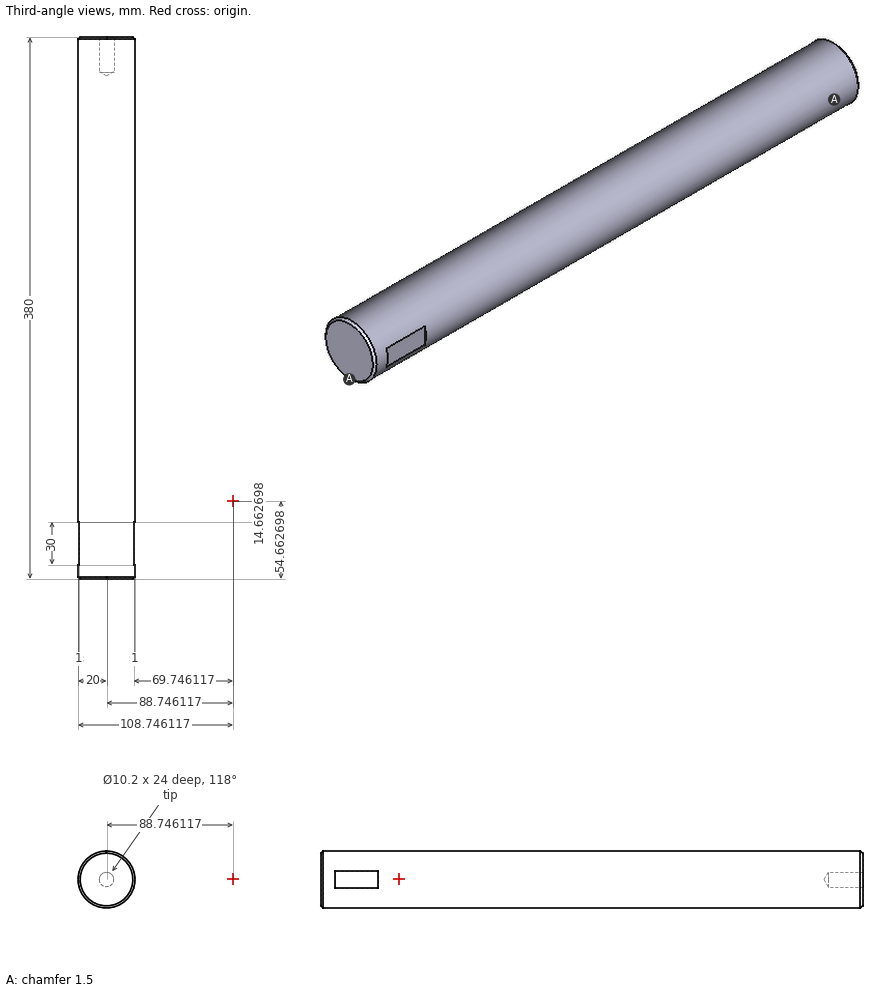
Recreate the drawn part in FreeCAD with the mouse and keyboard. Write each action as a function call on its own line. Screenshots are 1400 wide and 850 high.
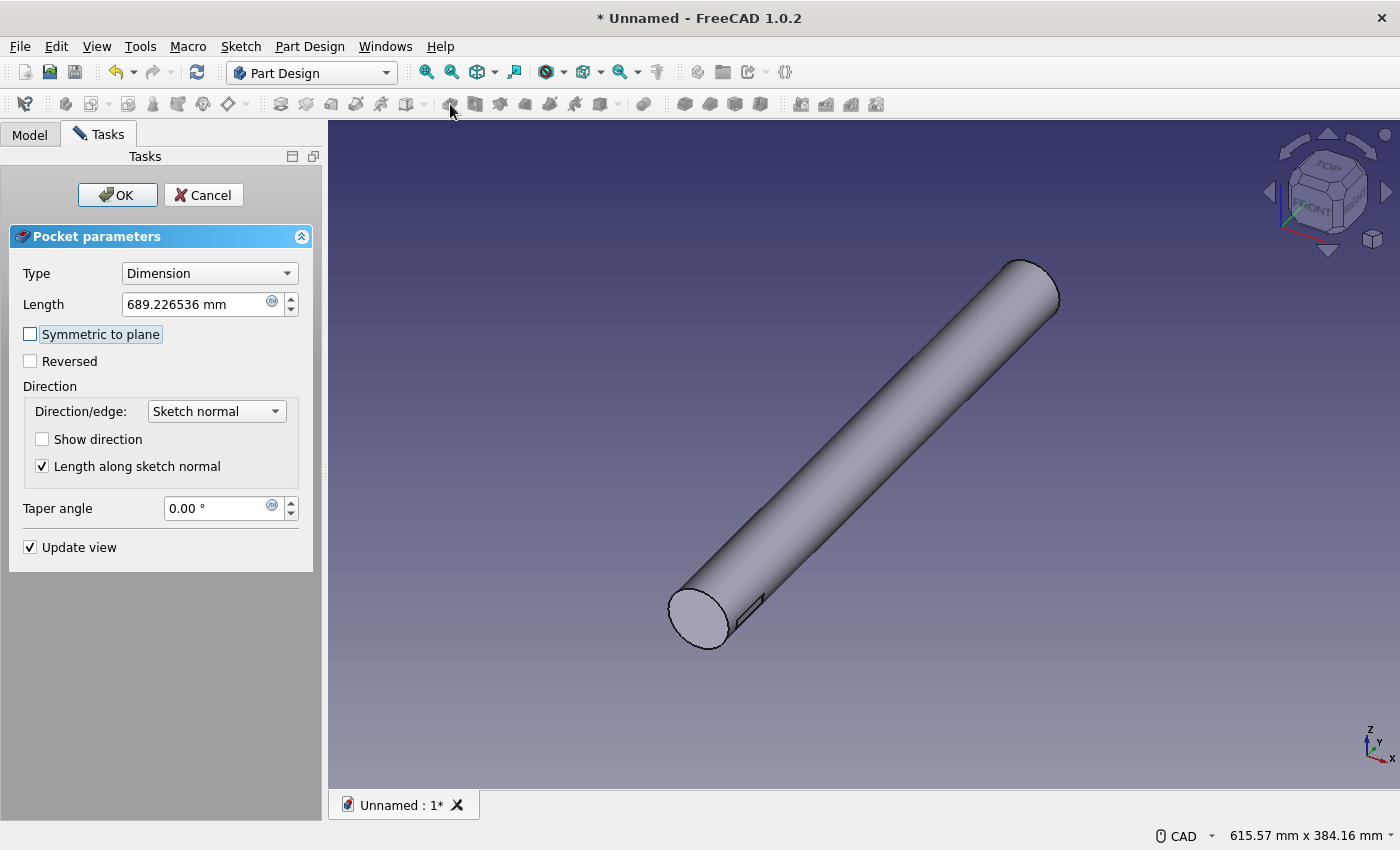
click(31, 334)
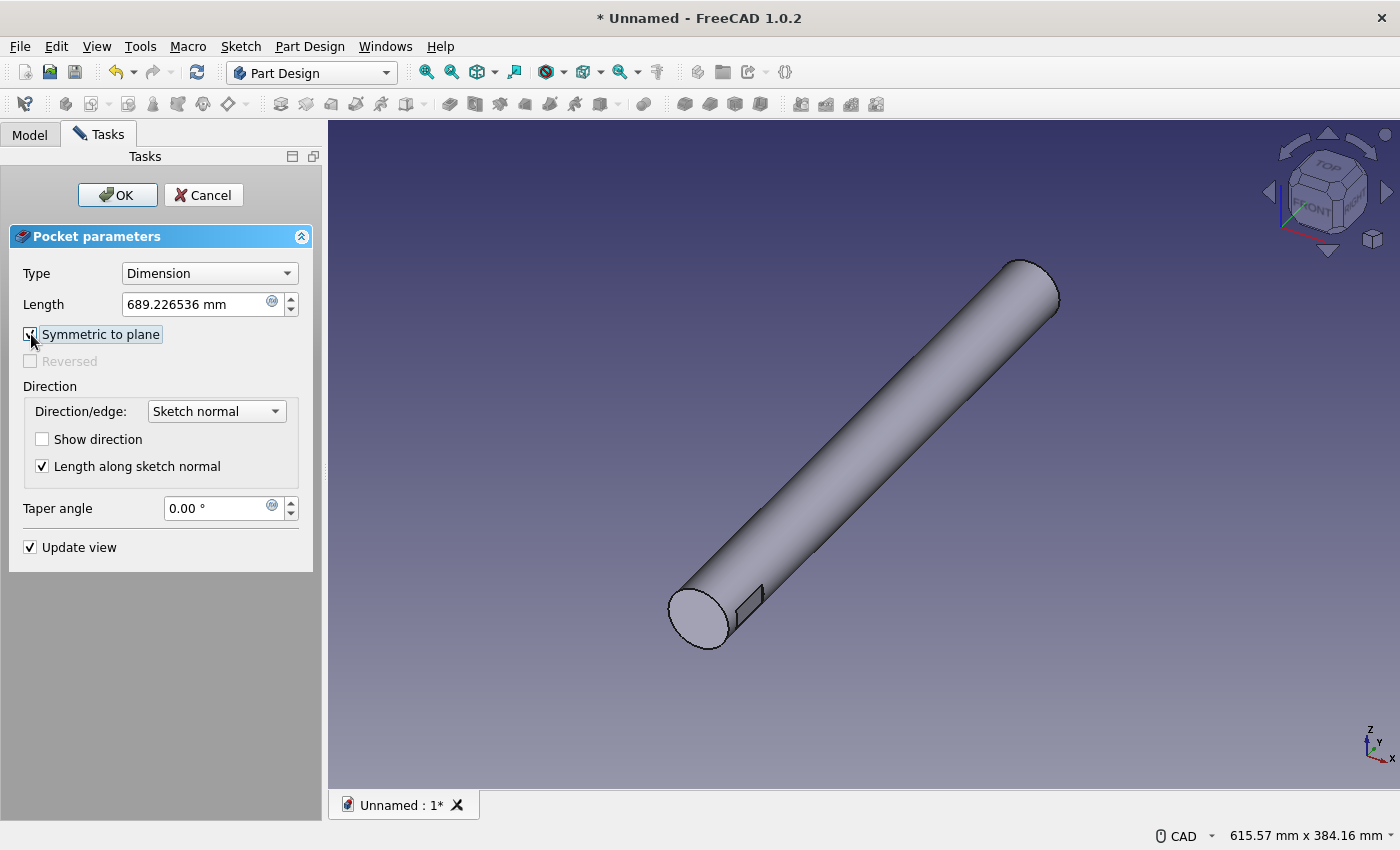
click(118, 195)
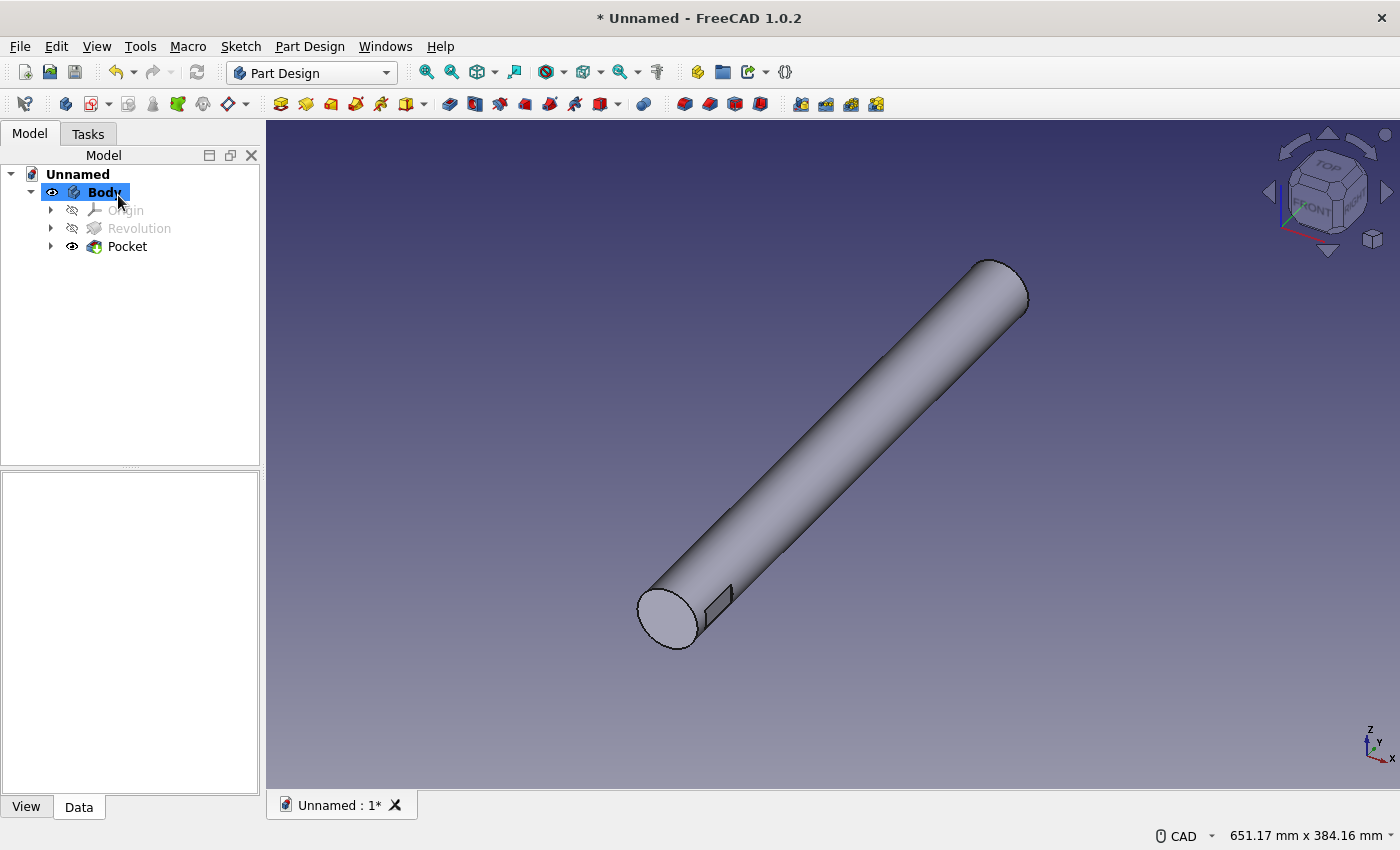
click(698, 628)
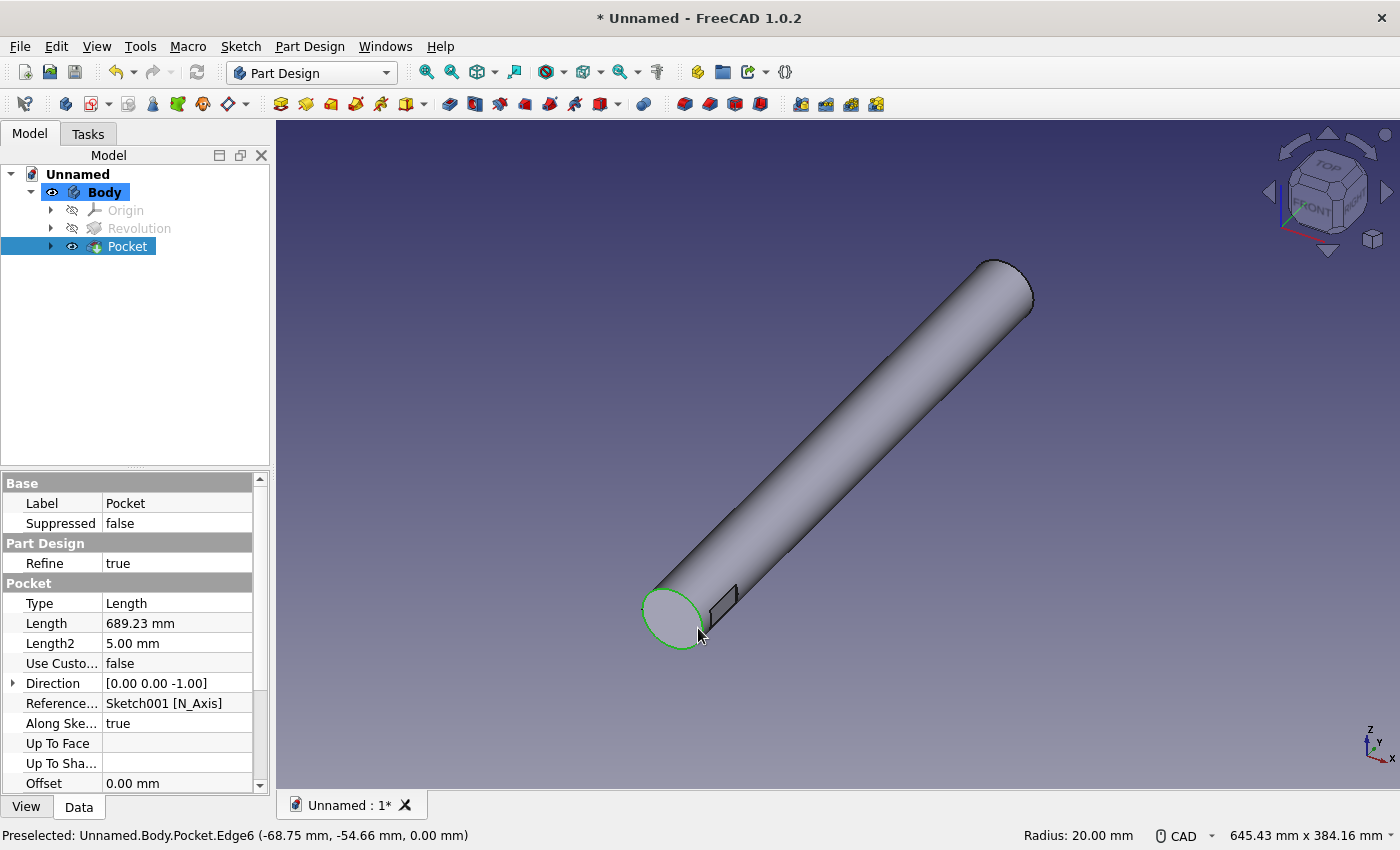
key(0)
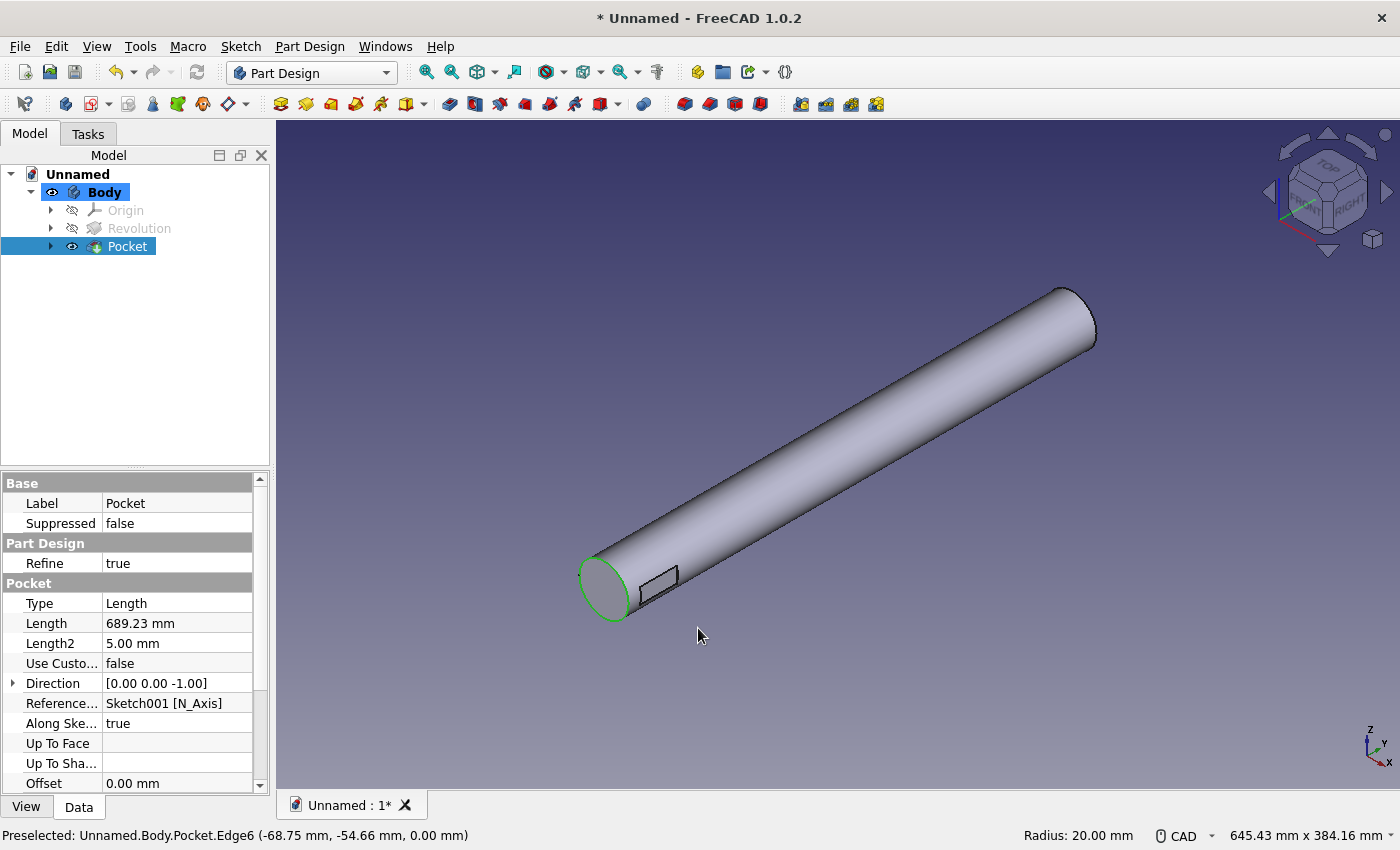
key(2)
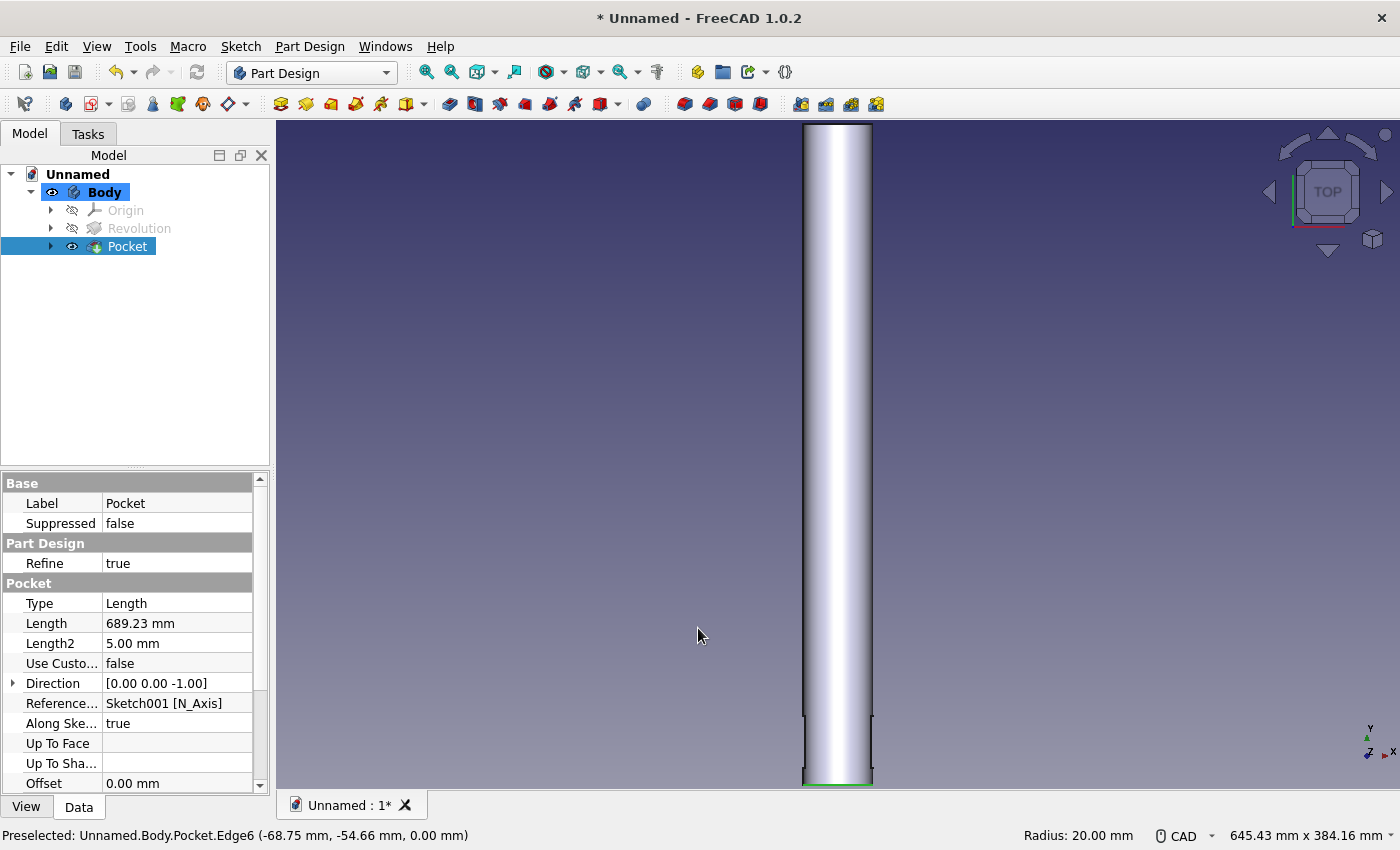
key(1)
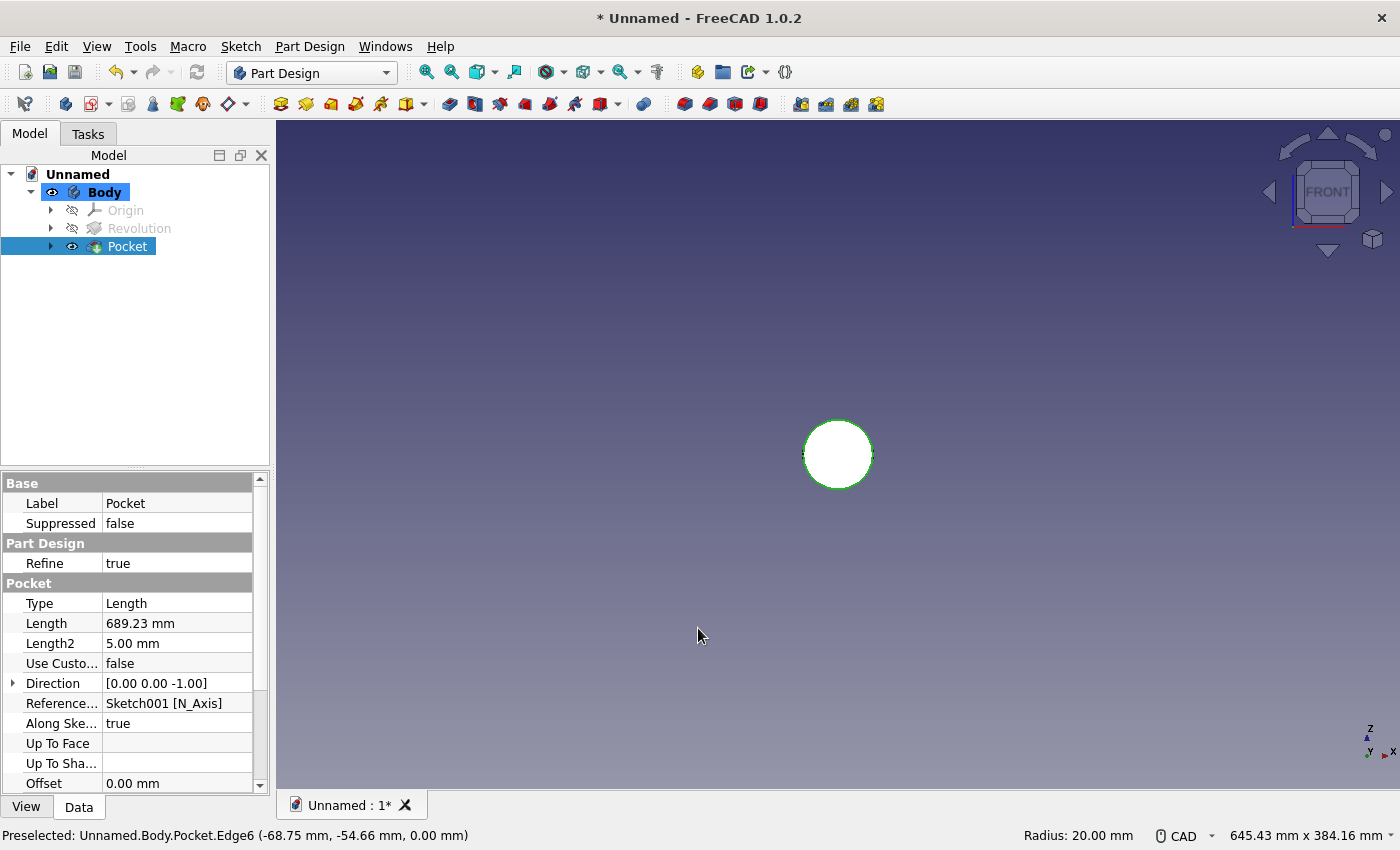
click(427, 72)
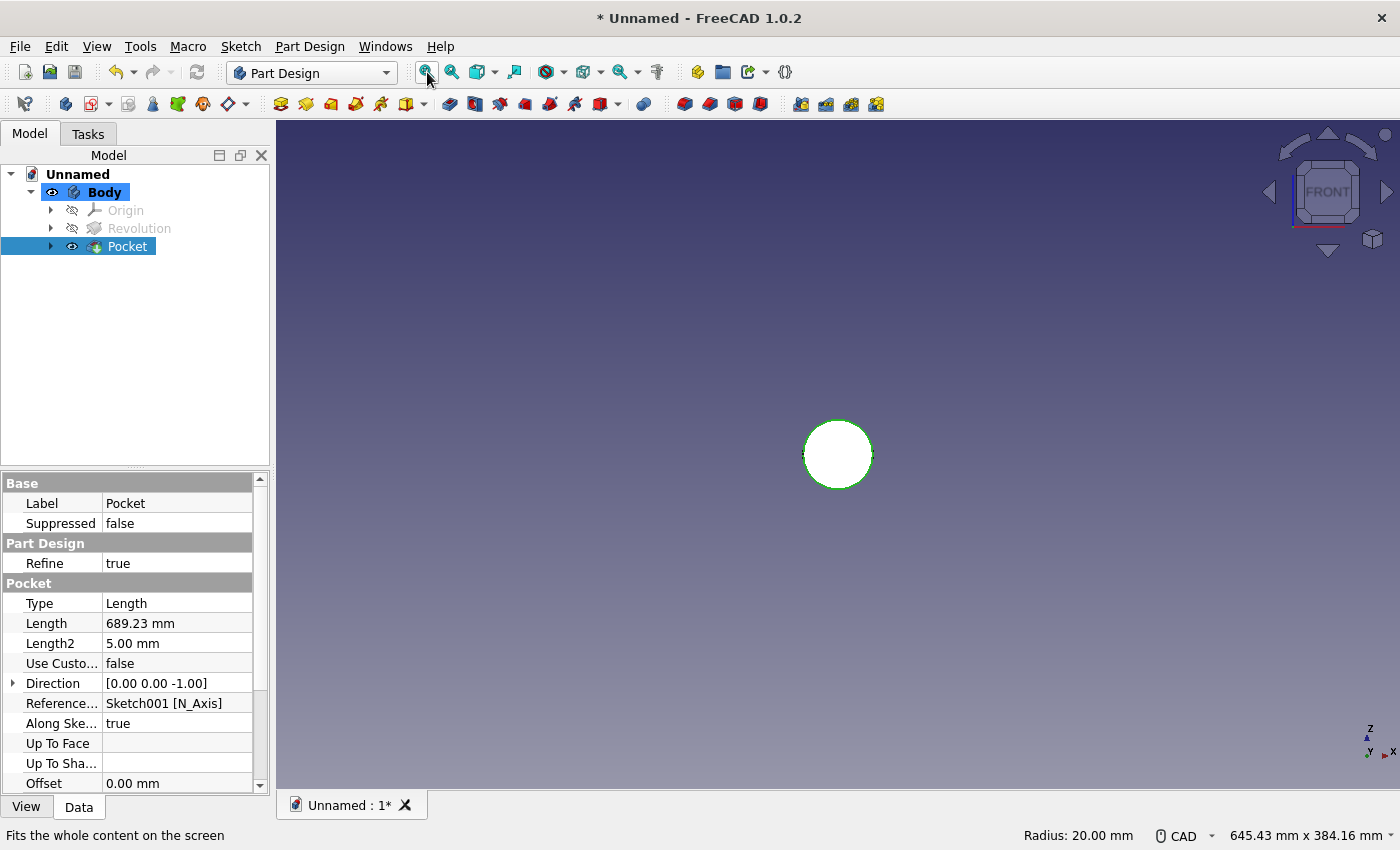
key(3)